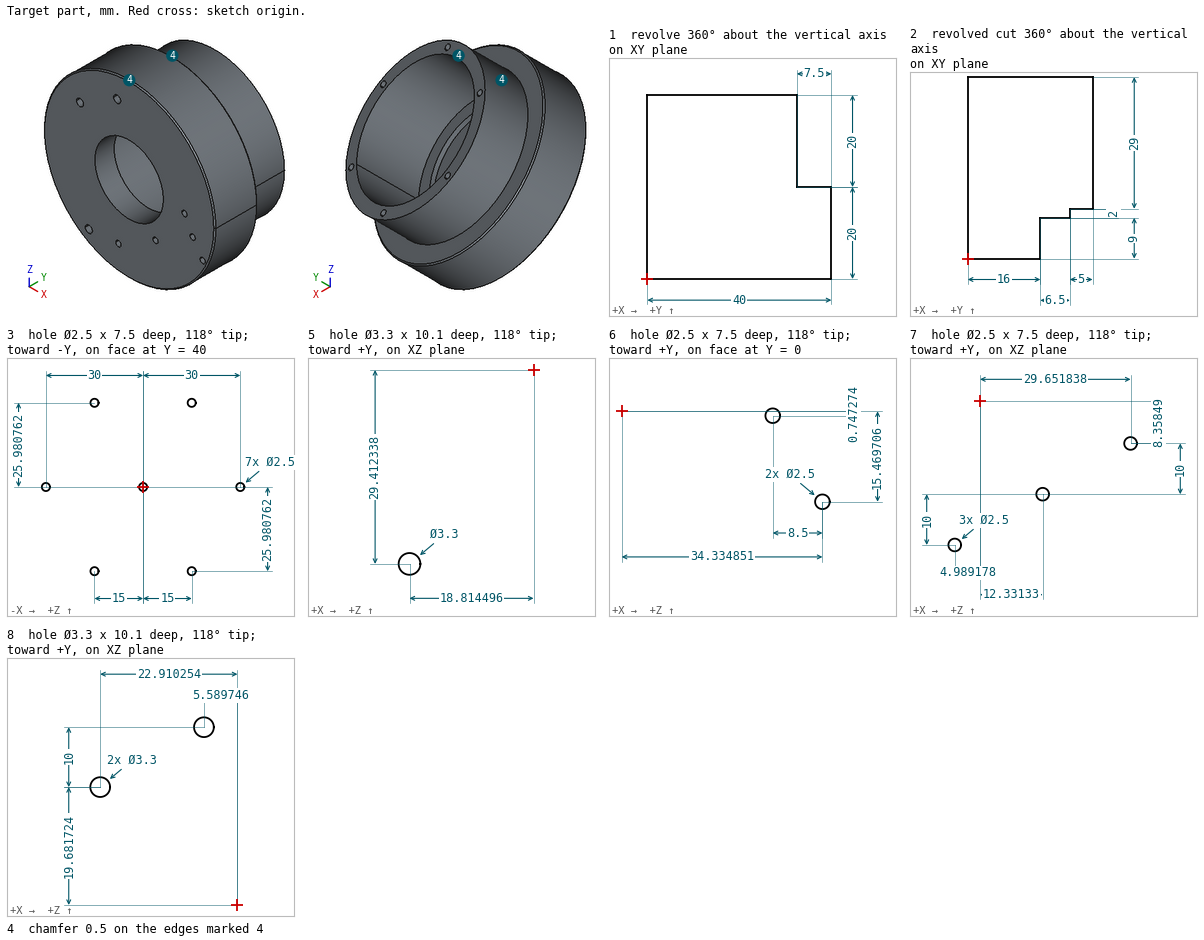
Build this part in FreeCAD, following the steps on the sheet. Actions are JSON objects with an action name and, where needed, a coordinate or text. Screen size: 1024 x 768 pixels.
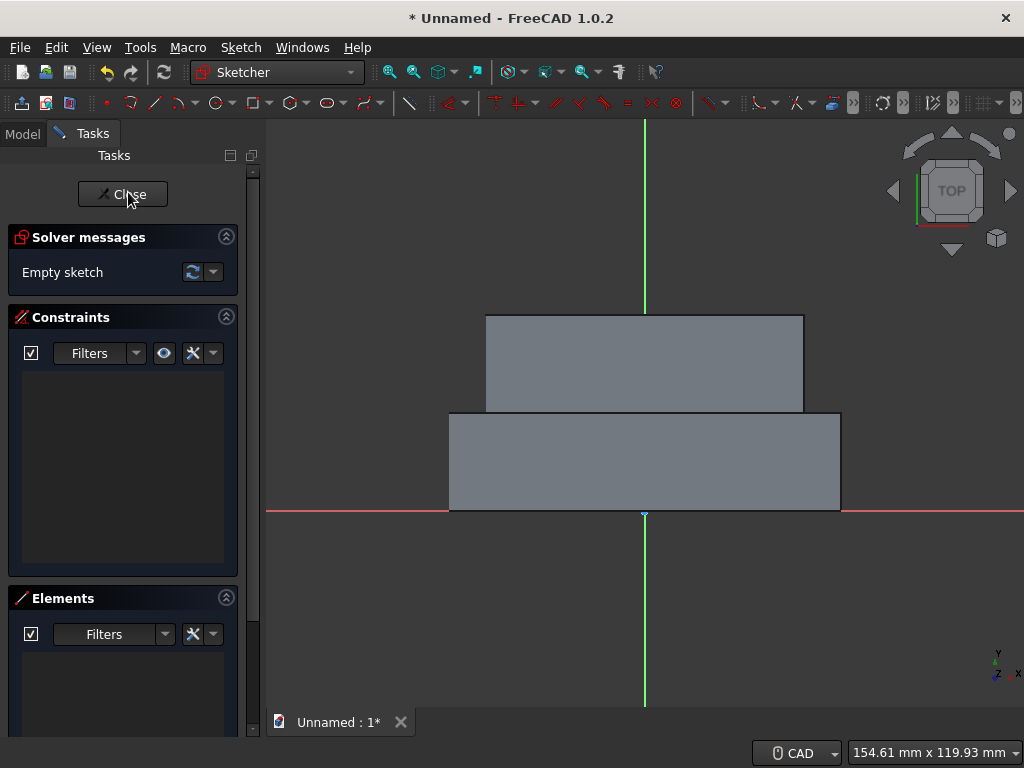
{"action": "left_click", "coordinate": [70, 104]}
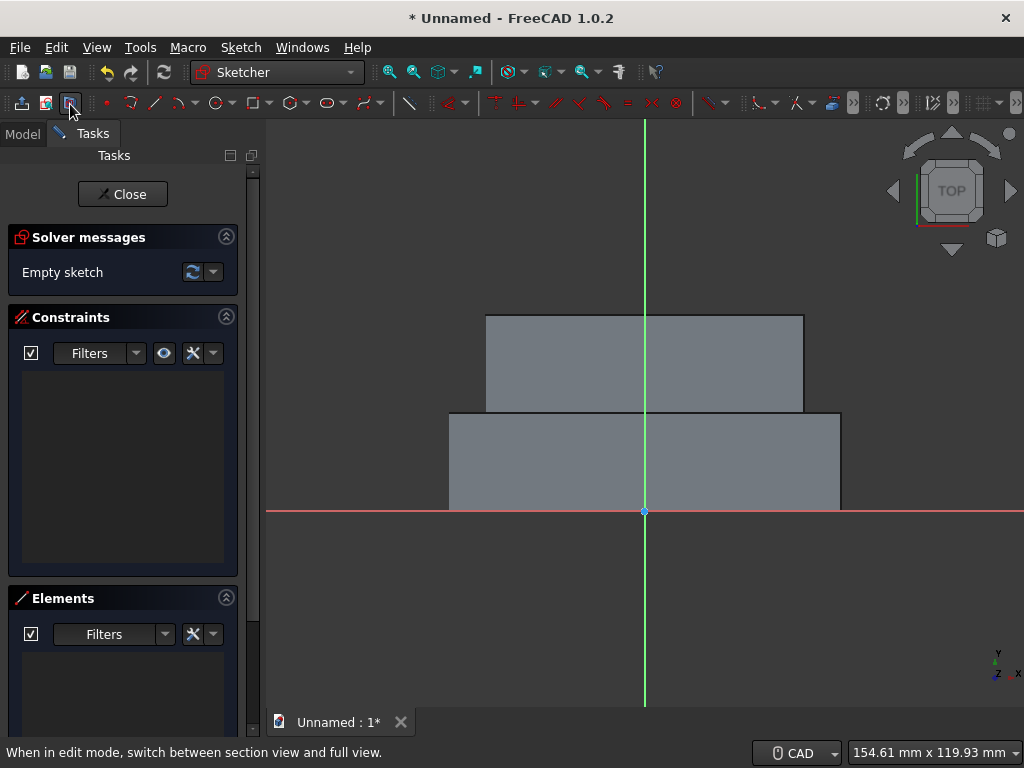
{"action": "scroll", "coordinate": [859, 413], "scroll_direction": "up", "scroll_amount": 3}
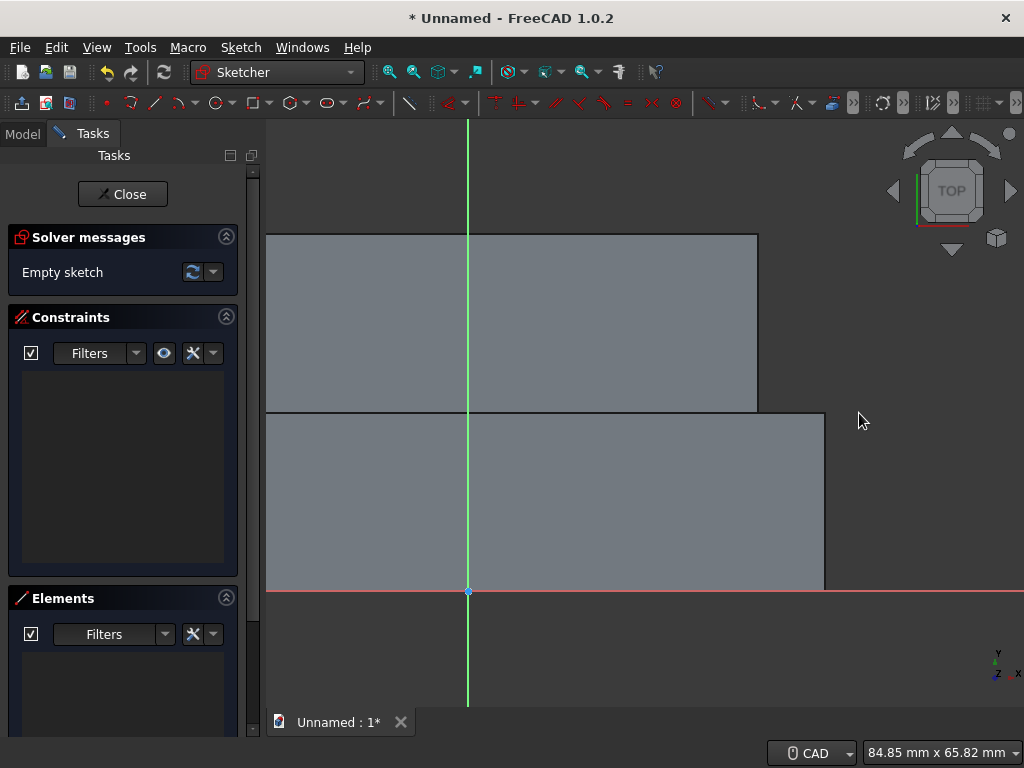
{"action": "left_click", "coordinate": [132, 104]}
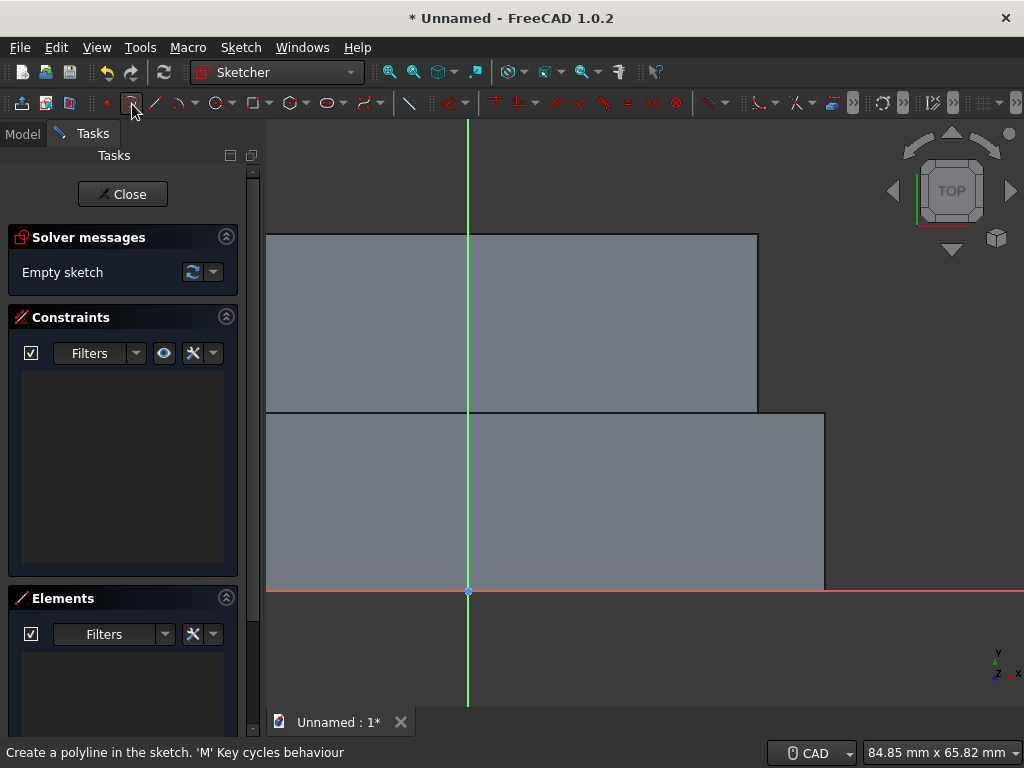
{"action": "left_click", "coordinate": [468, 591]}
{"action": "left_click", "coordinate": [611, 582]}
{"action": "left_click", "coordinate": [611, 511]}
{"action": "left_click", "coordinate": [669, 511]}
{"action": "left_click", "coordinate": [669, 493]}
{"action": "left_click", "coordinate": [714, 493]}
{"action": "left_click", "coordinate": [714, 234]}
{"action": "left_click", "coordinate": [477, 234]}
{"action": "left_click", "coordinate": [468, 591]}
{"action": "key", "text": "Escape"}
{"action": "key", "text": "Escape"}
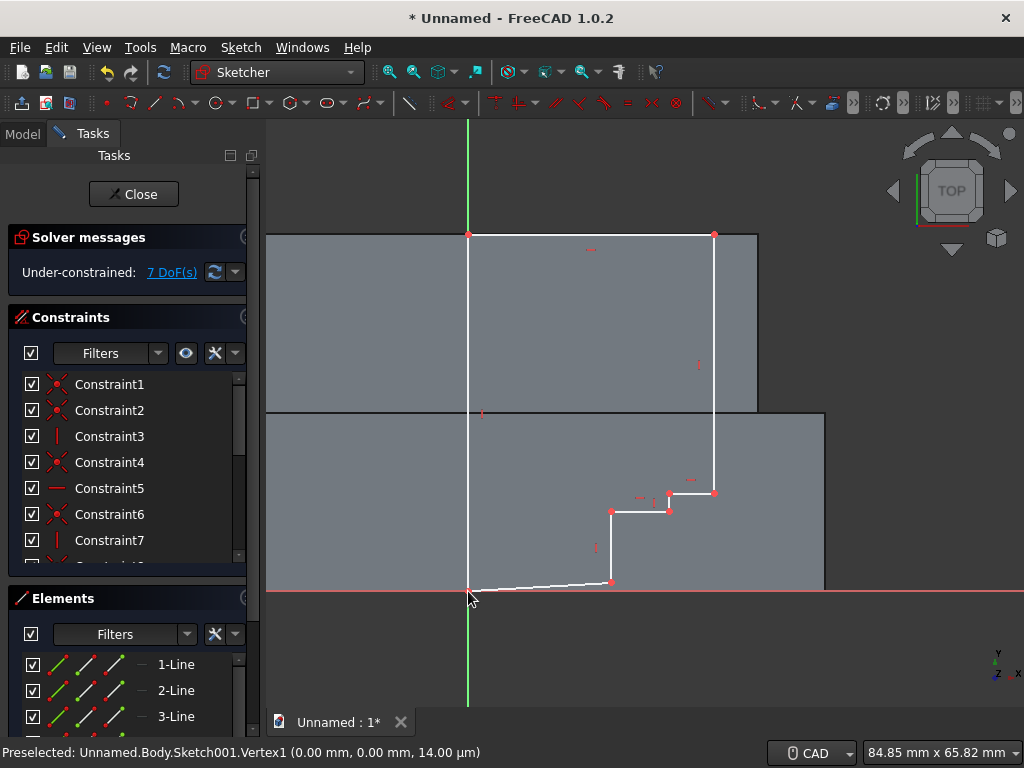
{"action": "left_click", "coordinate": [511, 589]}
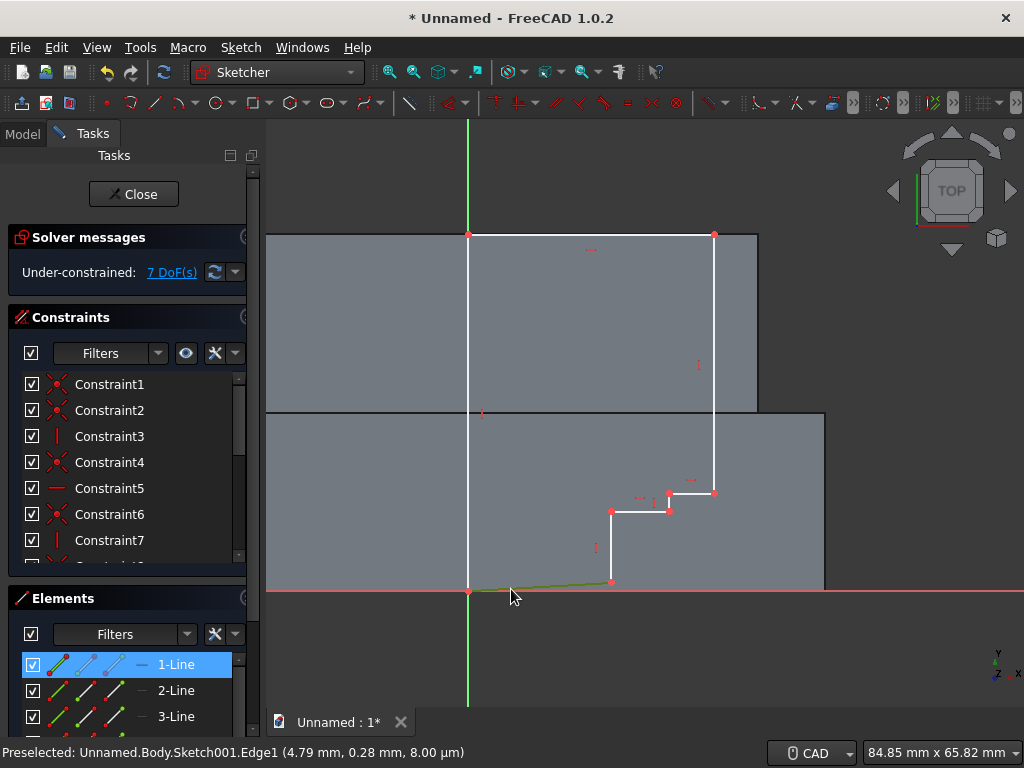
{"action": "left_click", "coordinate": [538, 104]}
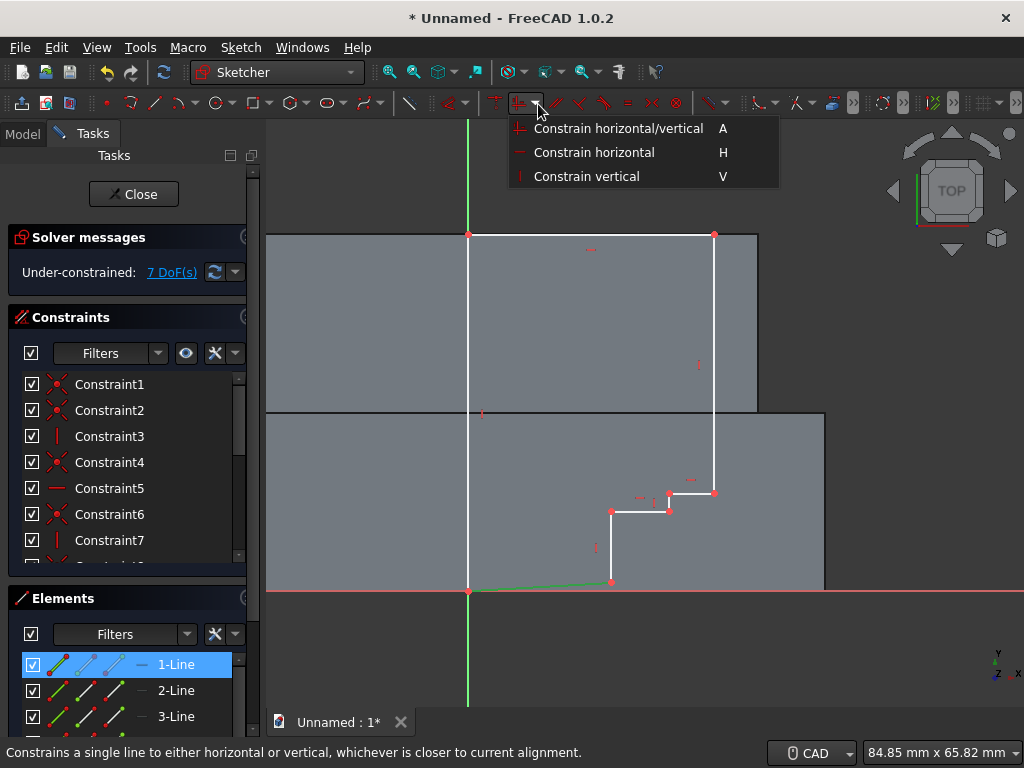
{"action": "left_click", "coordinate": [644, 152]}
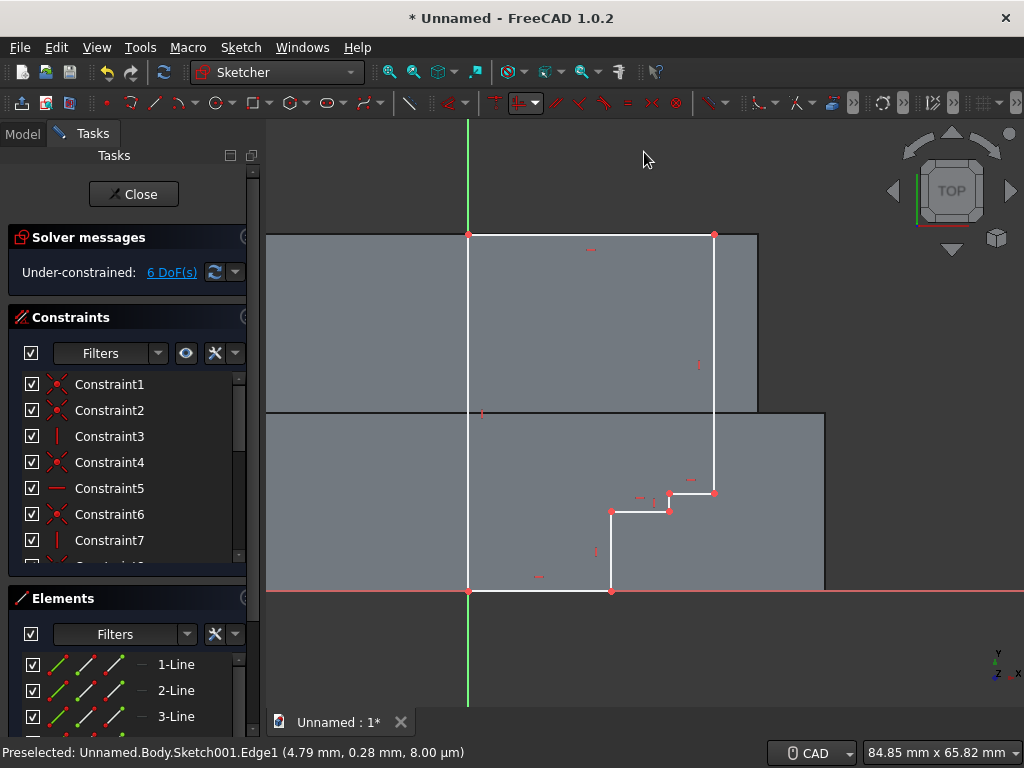
{"action": "left_click", "coordinate": [448, 104]}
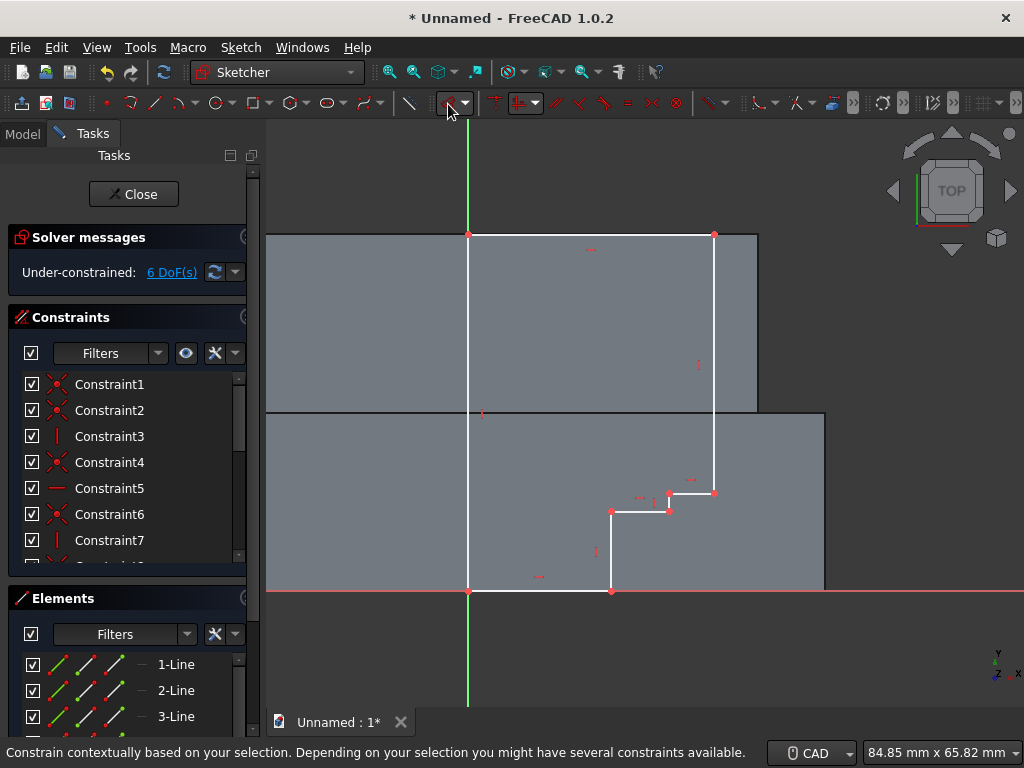
{"action": "left_click", "coordinate": [611, 567]}
{"action": "left_click", "coordinate": [645, 552]}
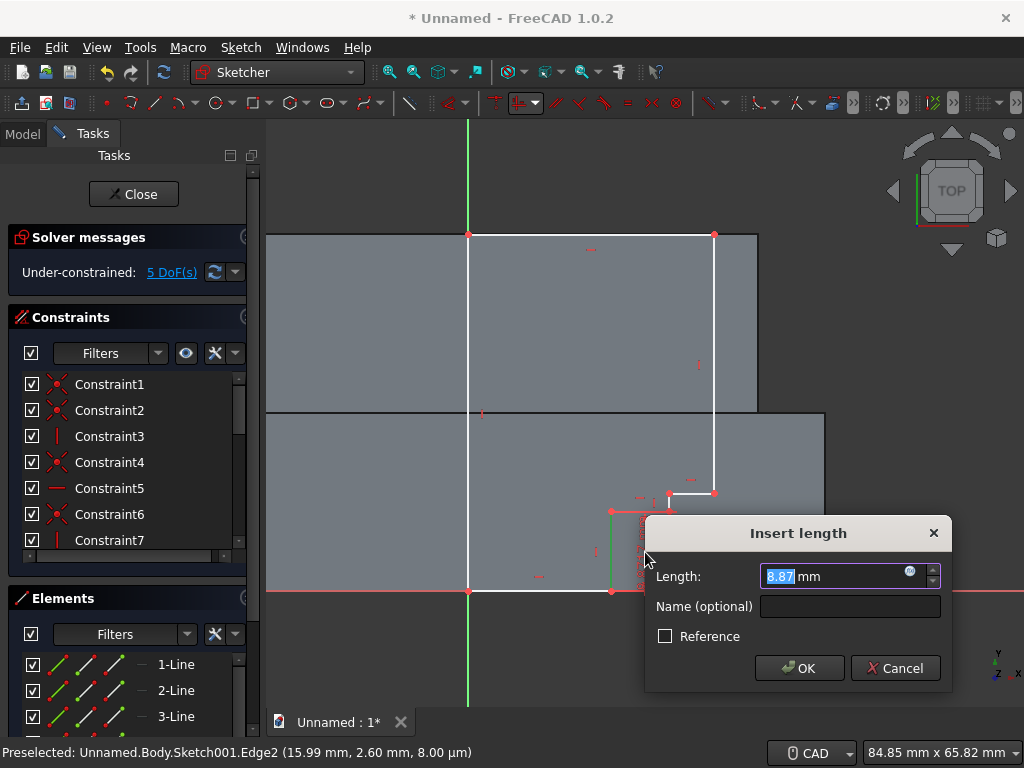
{"action": "type", "text": "9"}
{"action": "key", "text": "Return"}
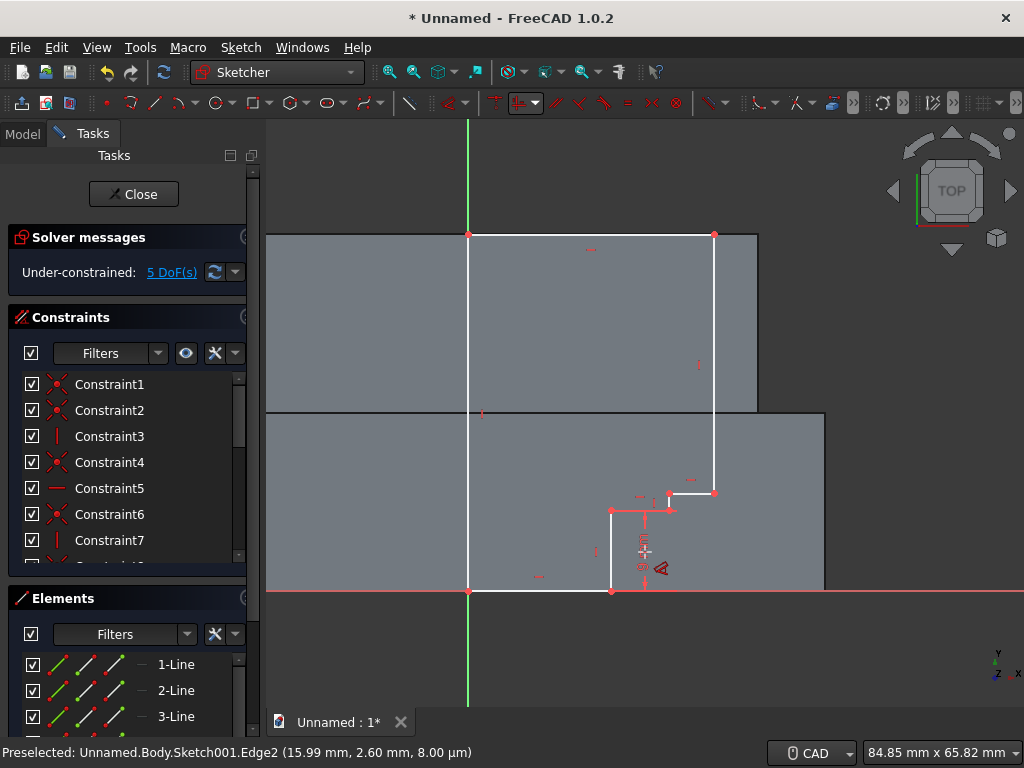
{"action": "scroll", "coordinate": [669, 502], "scroll_direction": "up", "scroll_amount": 4}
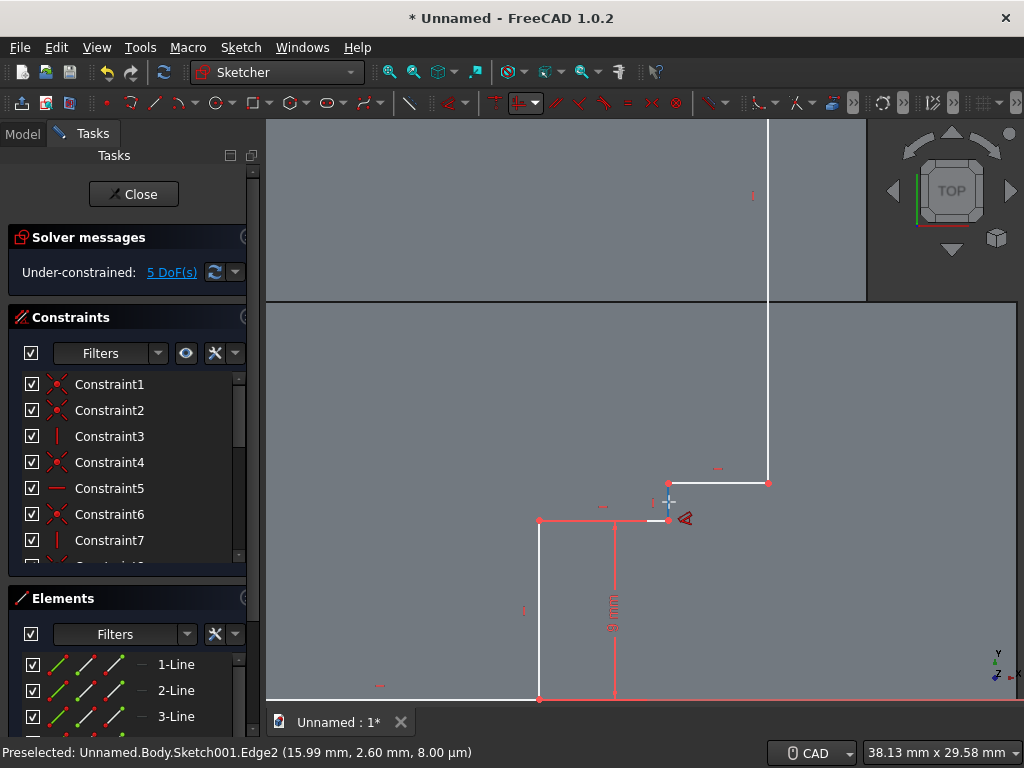
{"action": "left_click", "coordinate": [668, 502]}
{"action": "left_click", "coordinate": [702, 502]}